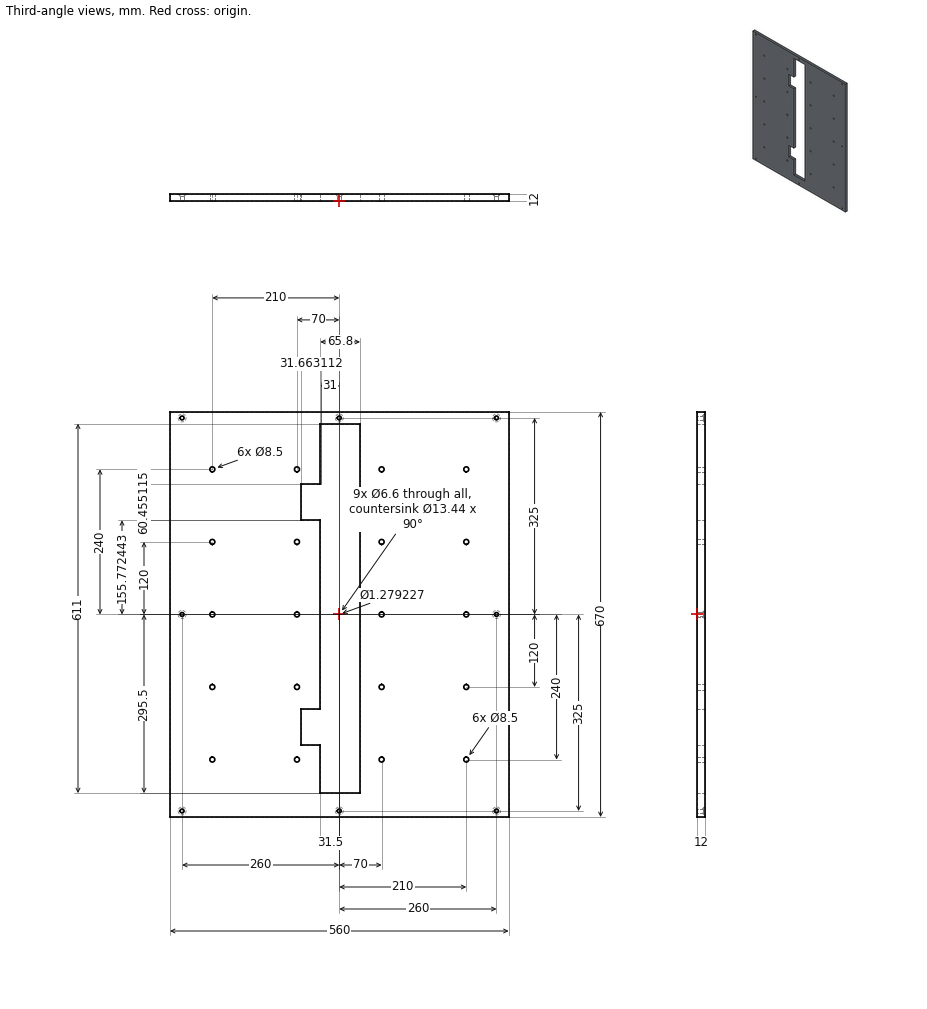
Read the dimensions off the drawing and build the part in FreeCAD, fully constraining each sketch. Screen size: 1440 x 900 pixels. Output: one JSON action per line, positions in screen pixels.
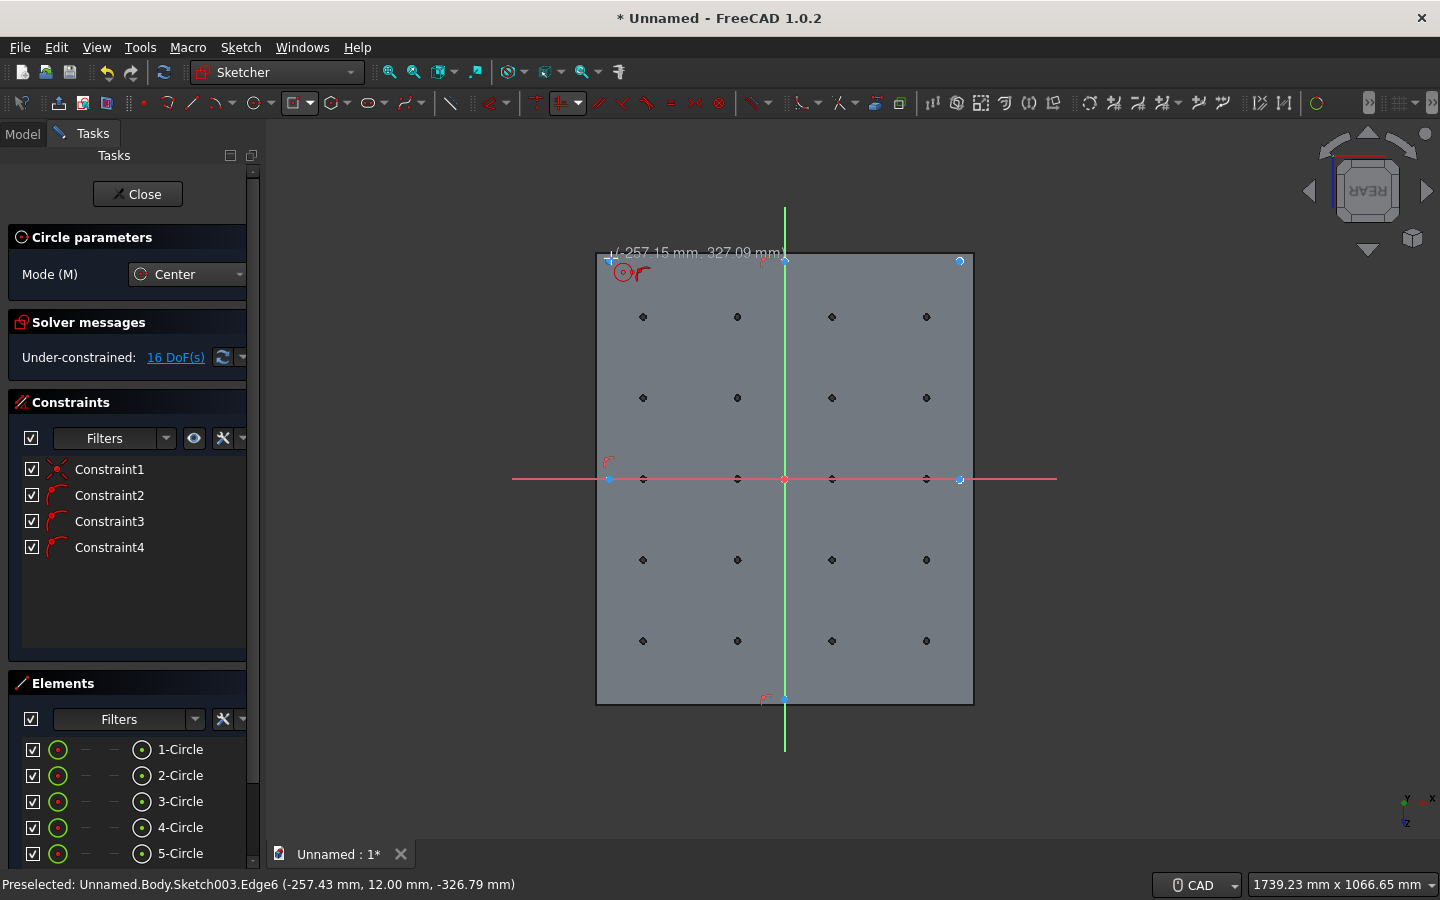
{"action": "scroll", "coordinate": [609, 698], "scroll_direction": "up", "scroll_amount": 12}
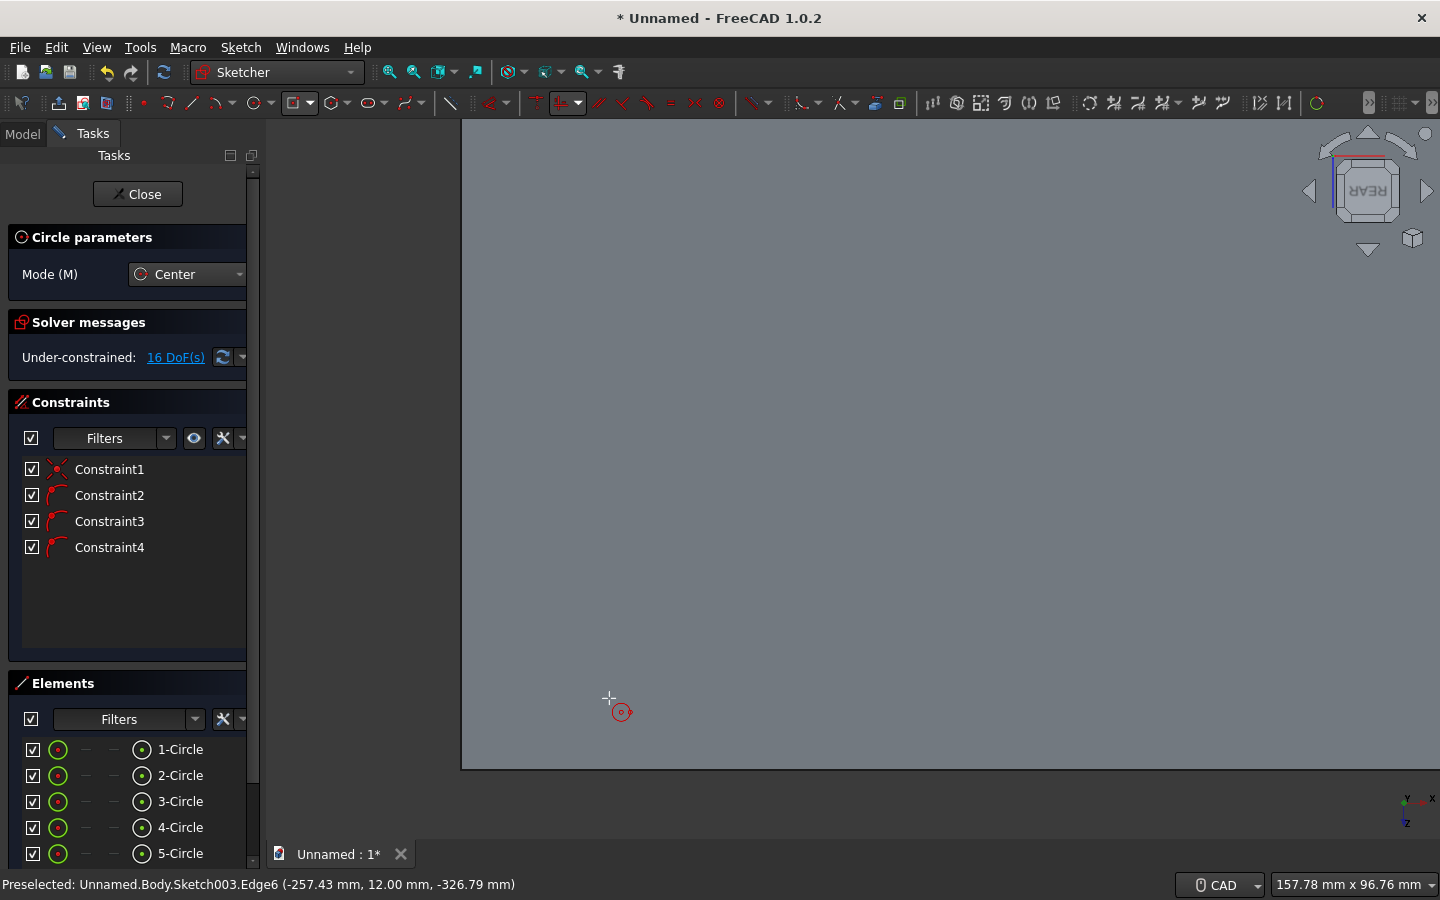
{"action": "scroll", "coordinate": [609, 699], "scroll_direction": "down", "scroll_amount": 12}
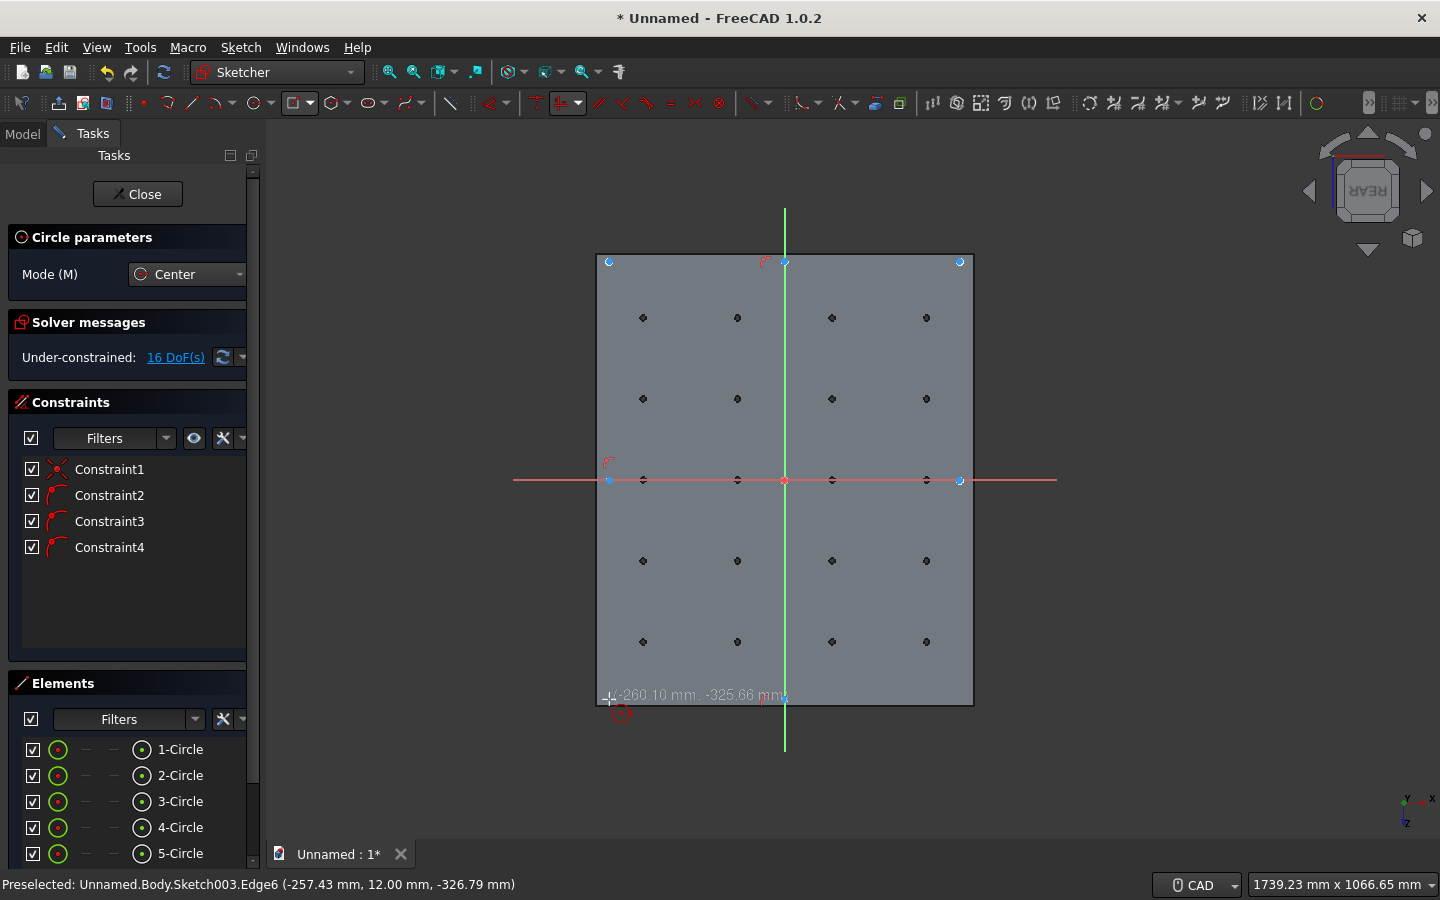
{"action": "left_click", "coordinate": [609, 699]}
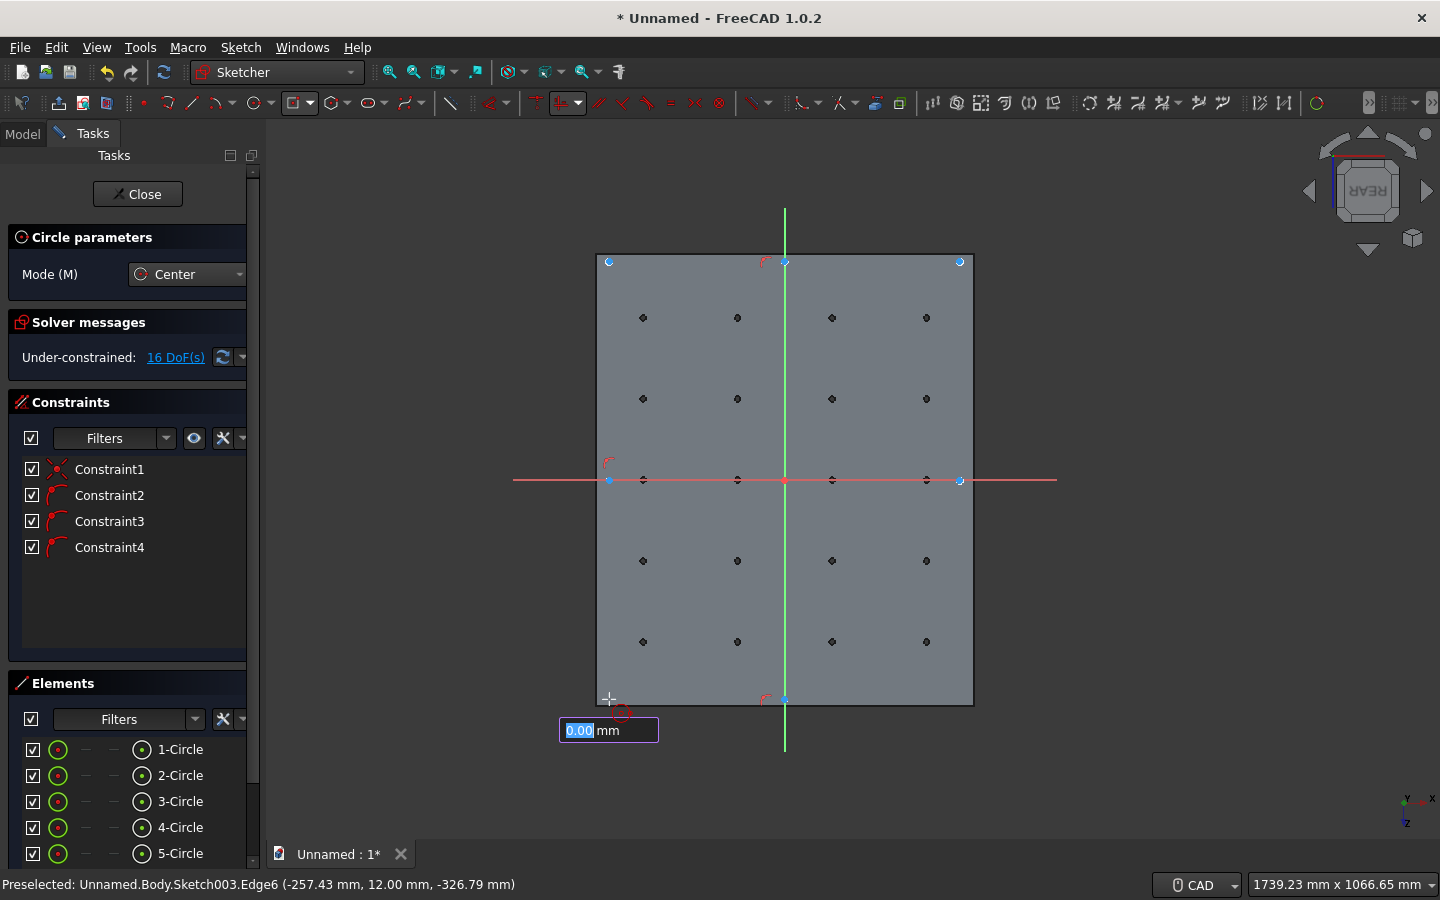
{"action": "scroll", "coordinate": [611, 698], "scroll_direction": "up", "scroll_amount": 10}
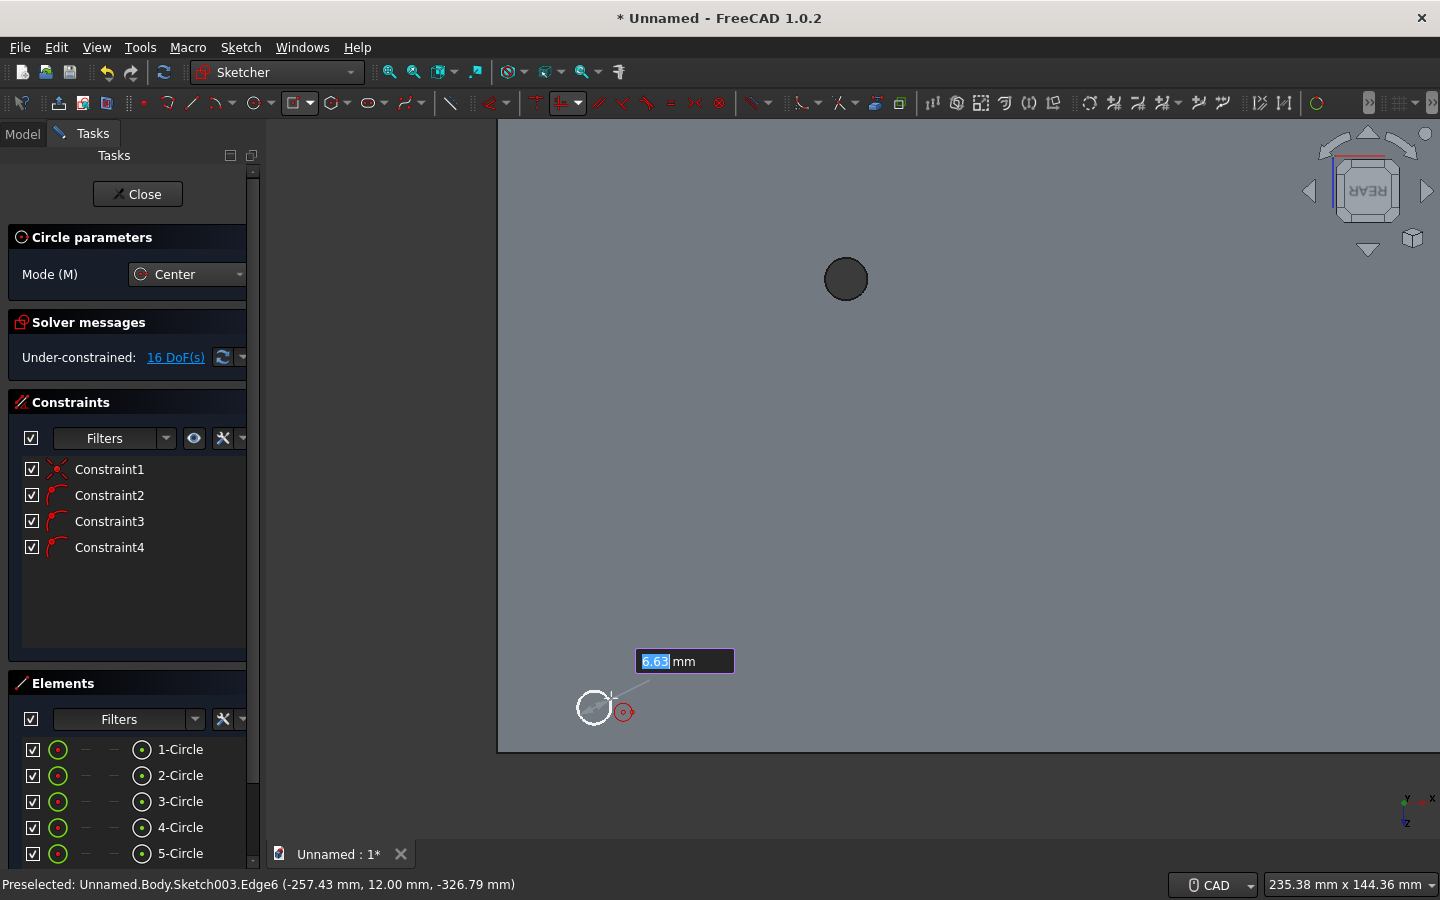
{"action": "left_click", "coordinate": [608, 691]}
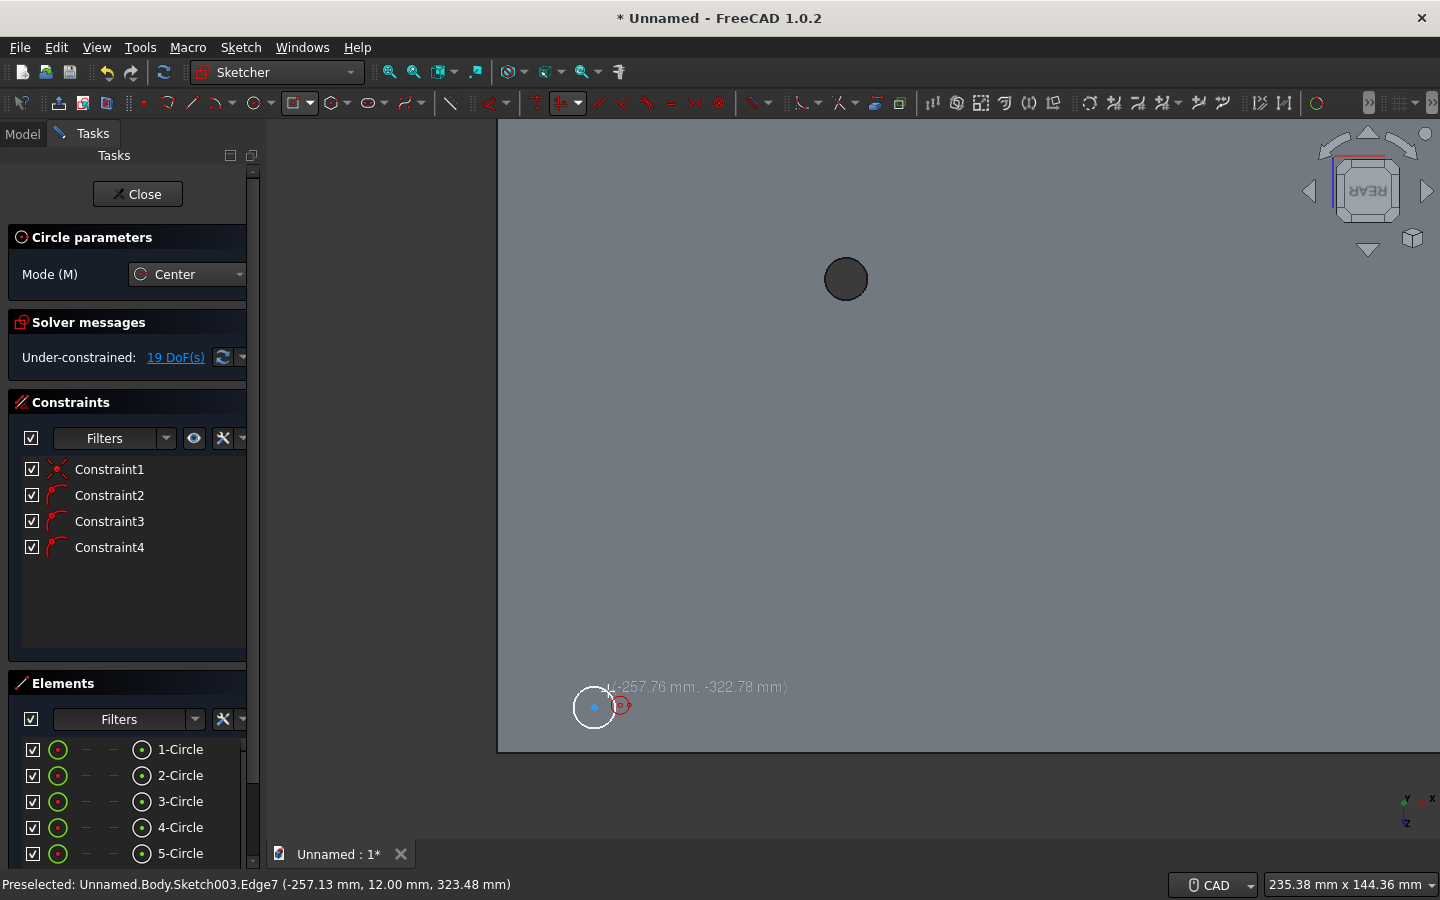
{"action": "scroll", "coordinate": [611, 698], "scroll_direction": "down", "scroll_amount": 10}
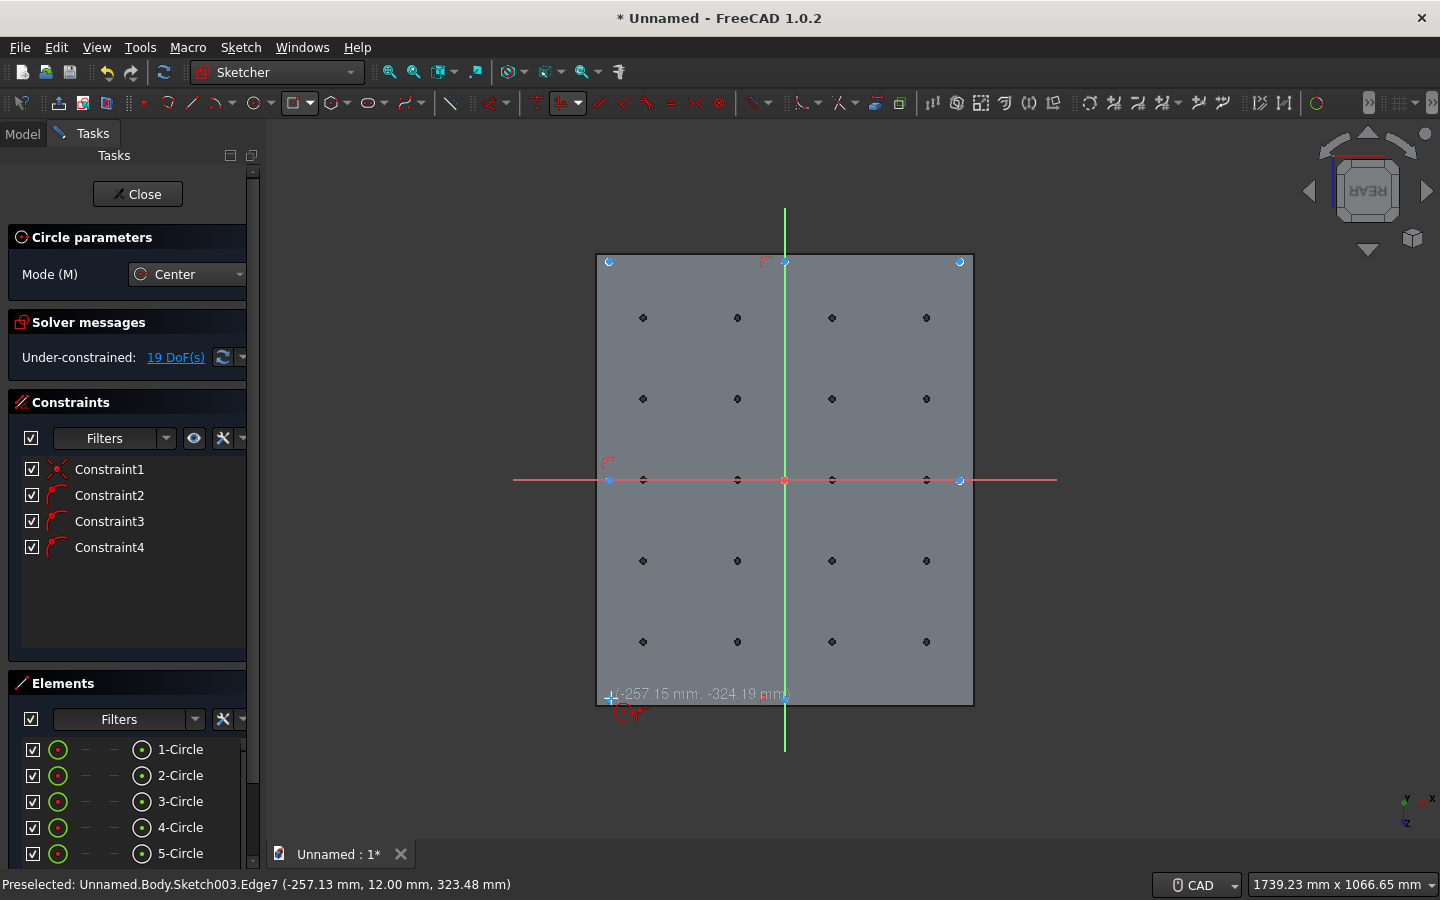
{"action": "scroll", "coordinate": [960, 699], "scroll_direction": "up", "scroll_amount": 12}